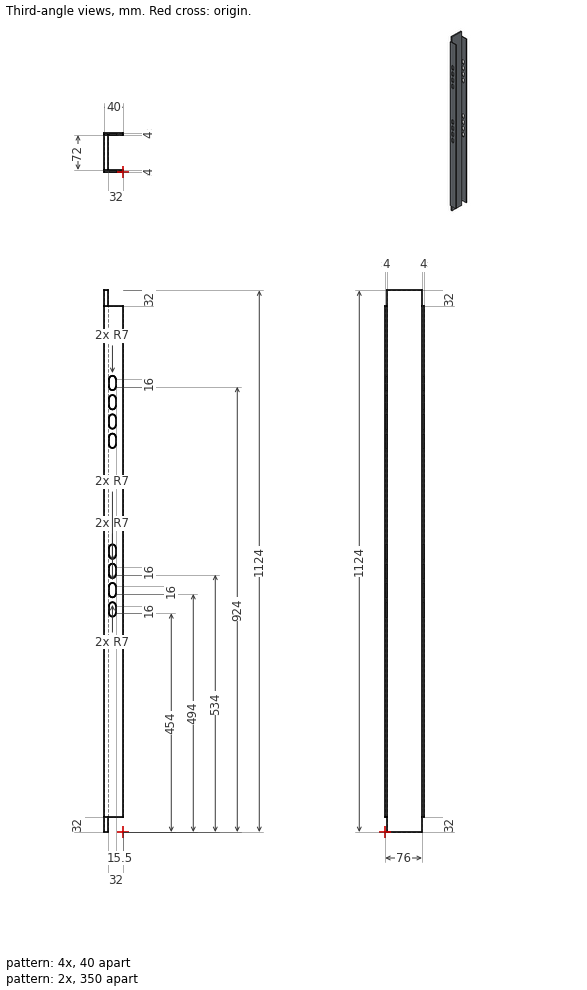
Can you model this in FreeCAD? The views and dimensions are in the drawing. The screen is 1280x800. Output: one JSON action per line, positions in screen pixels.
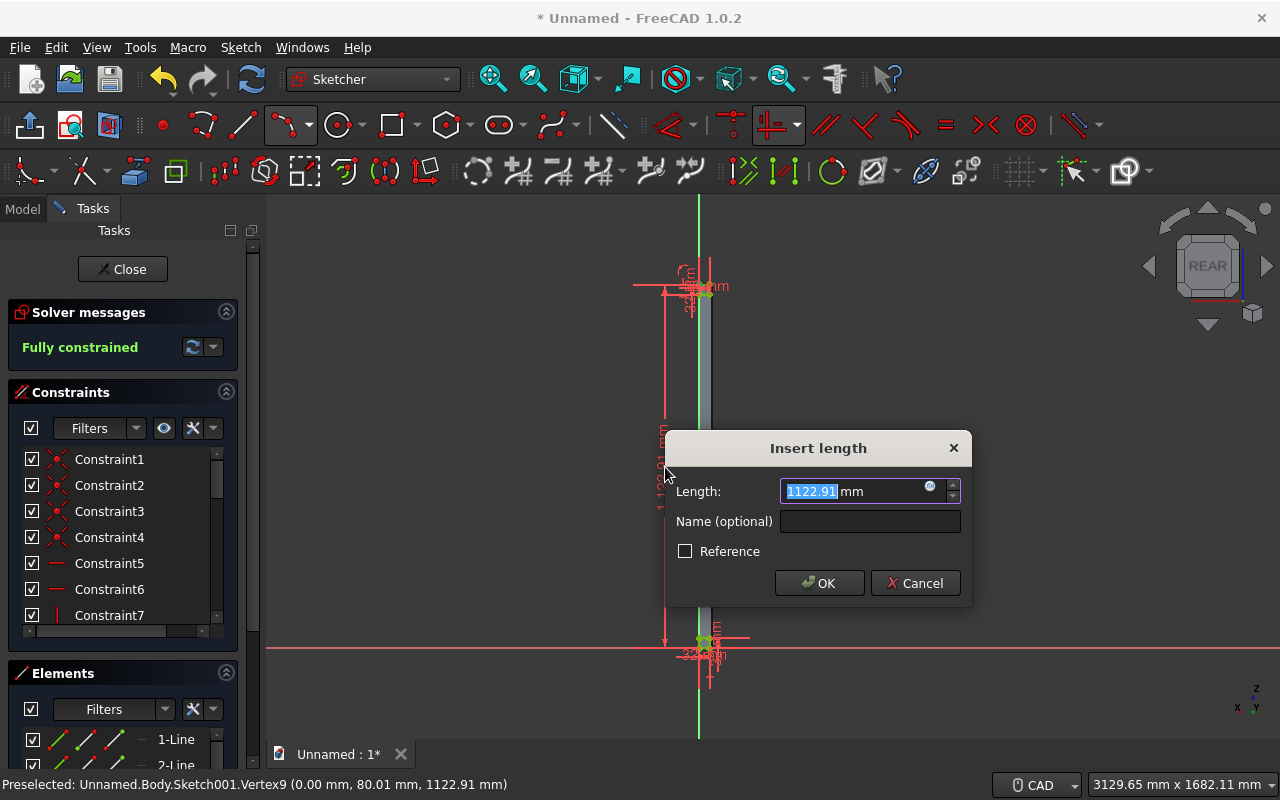
{"action": "type", "text": "1124"}
{"action": "key", "text": "Return"}
{"action": "key", "text": "Escape"}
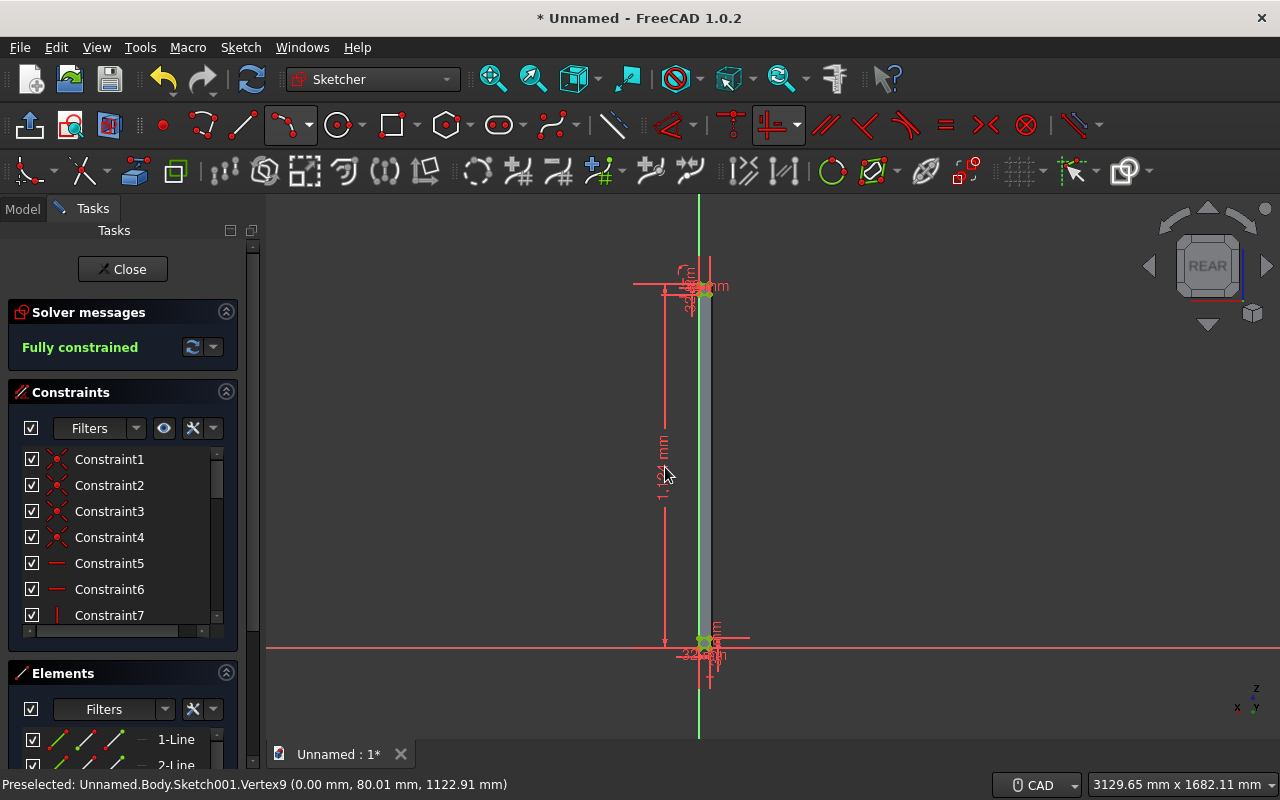
{"action": "left_click", "coordinate": [123, 269]}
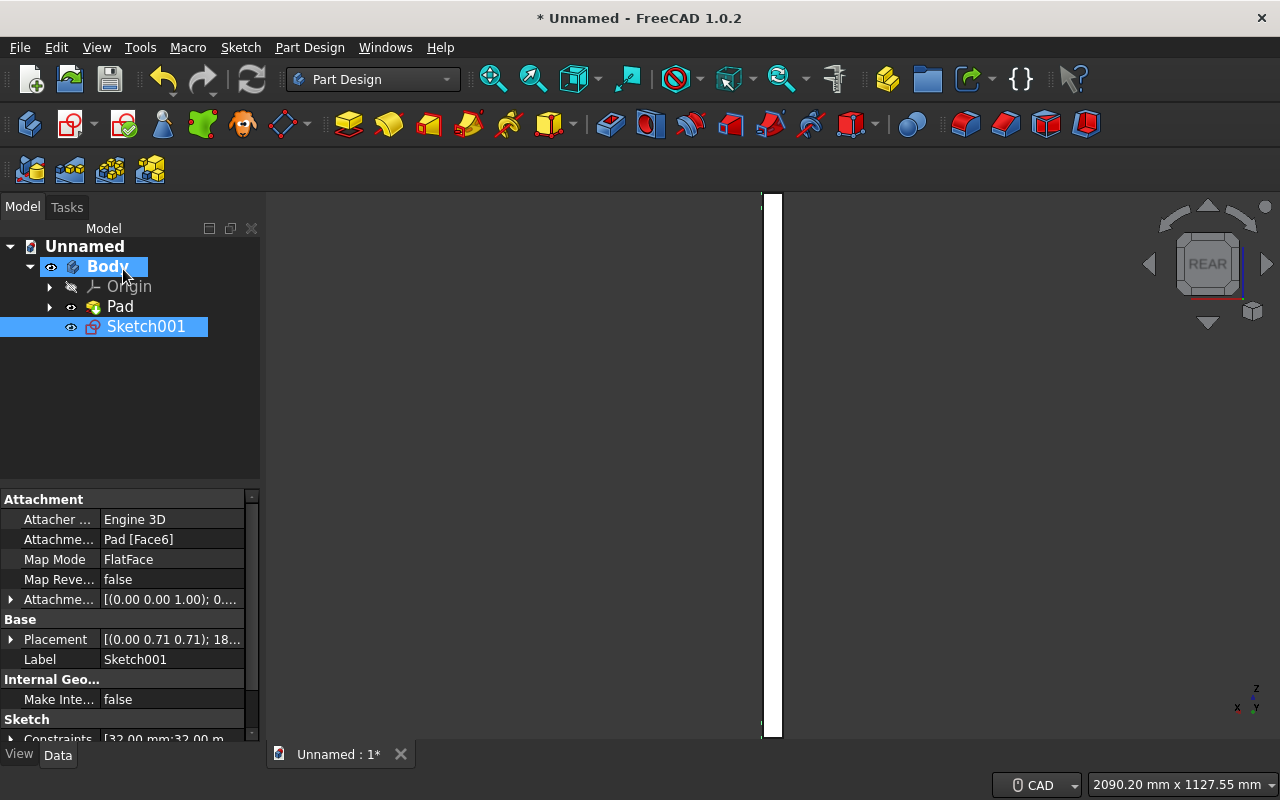
{"action": "left_click", "coordinate": [612, 124]}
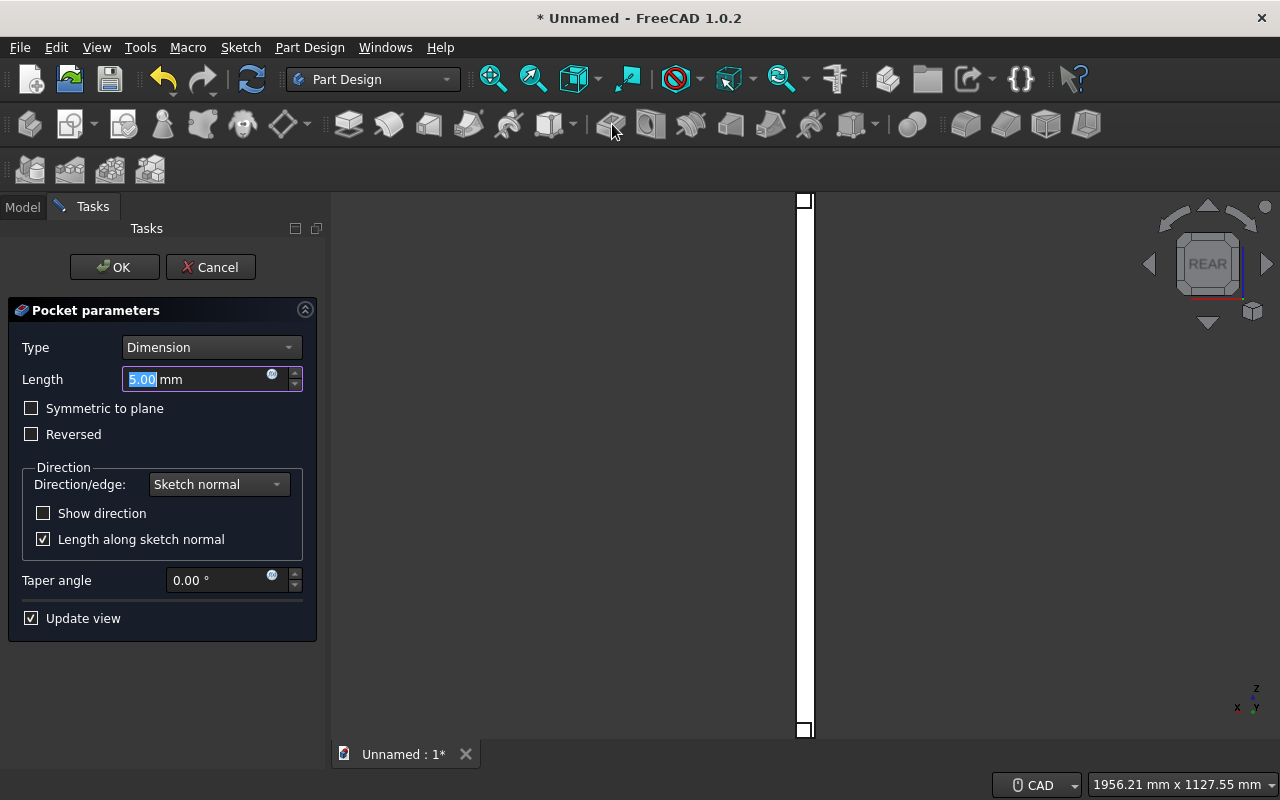
{"action": "left_click", "coordinate": [212, 348]}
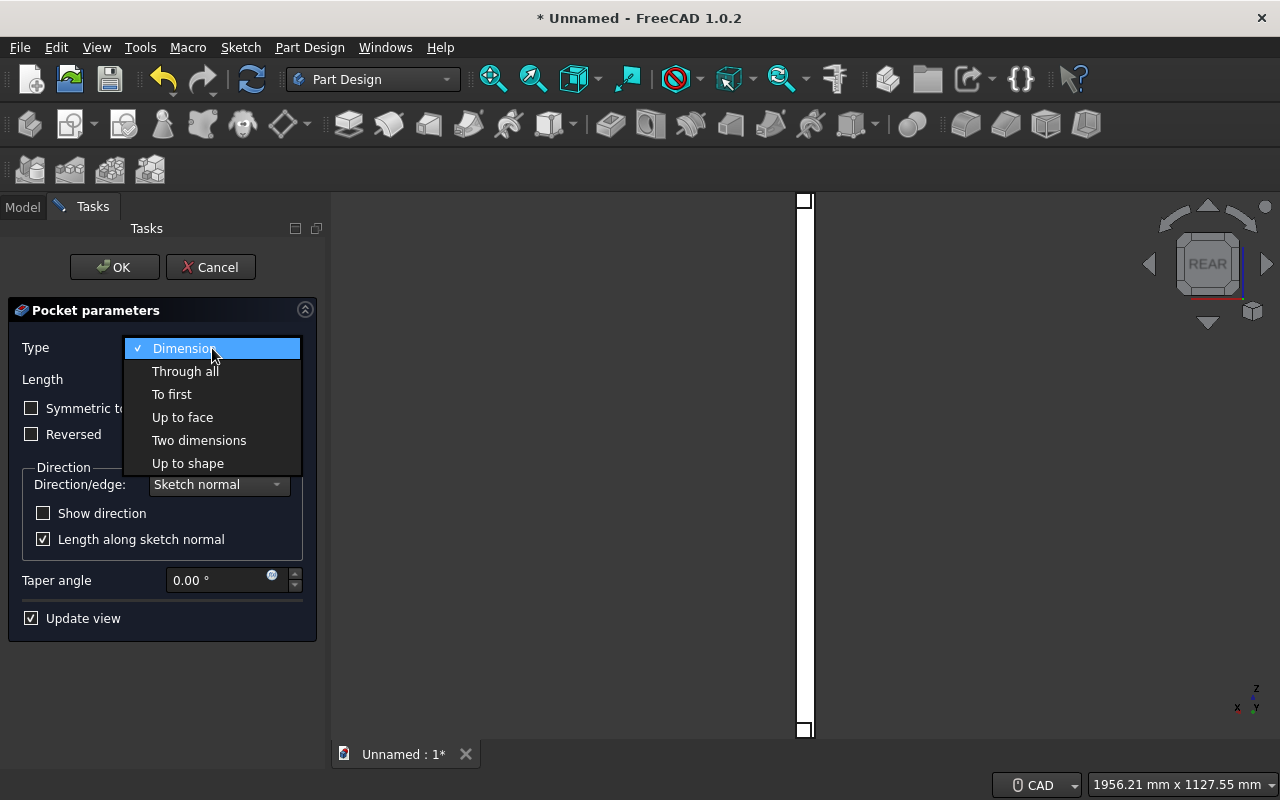
{"action": "left_click", "coordinate": [212, 372]}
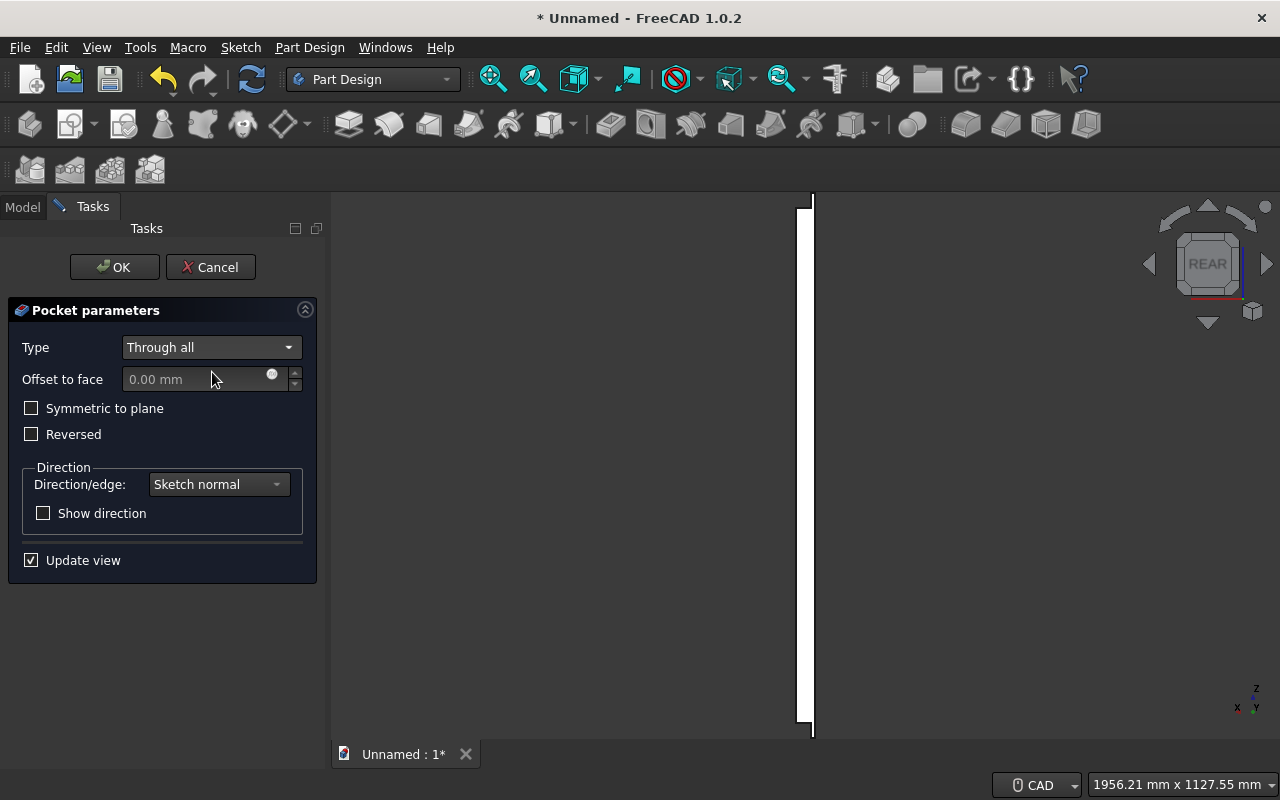
{"action": "left_click", "coordinate": [115, 267]}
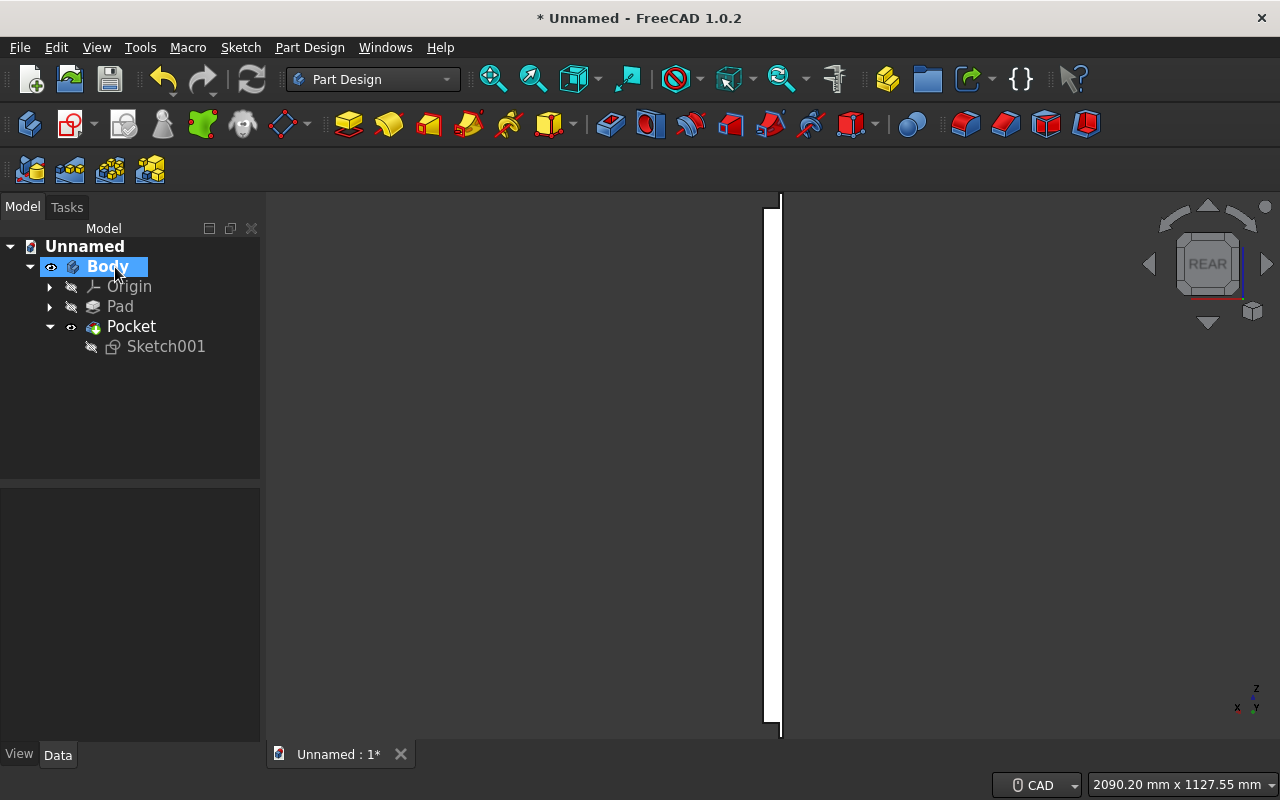
{"action": "key", "text": "0"}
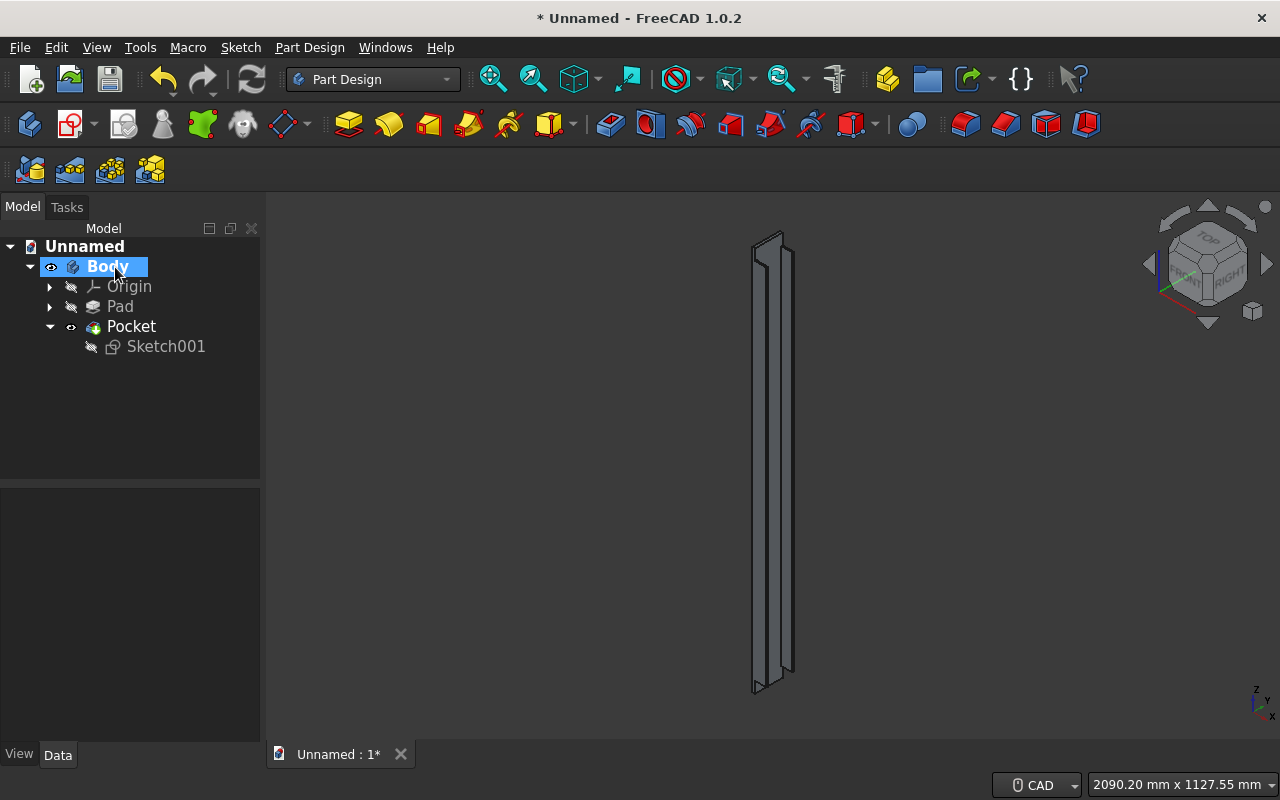
{"action": "key", "text": "3"}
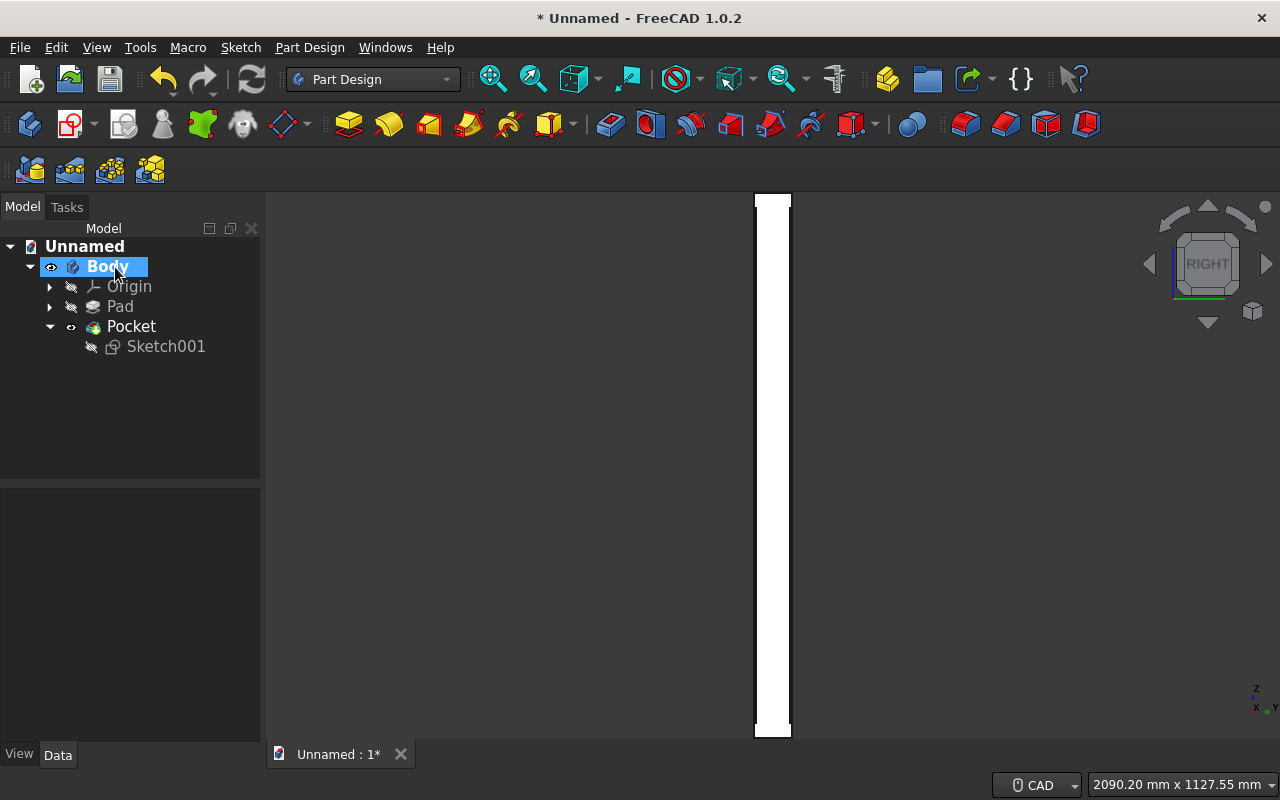
{"action": "left_click", "coordinate": [773, 231]}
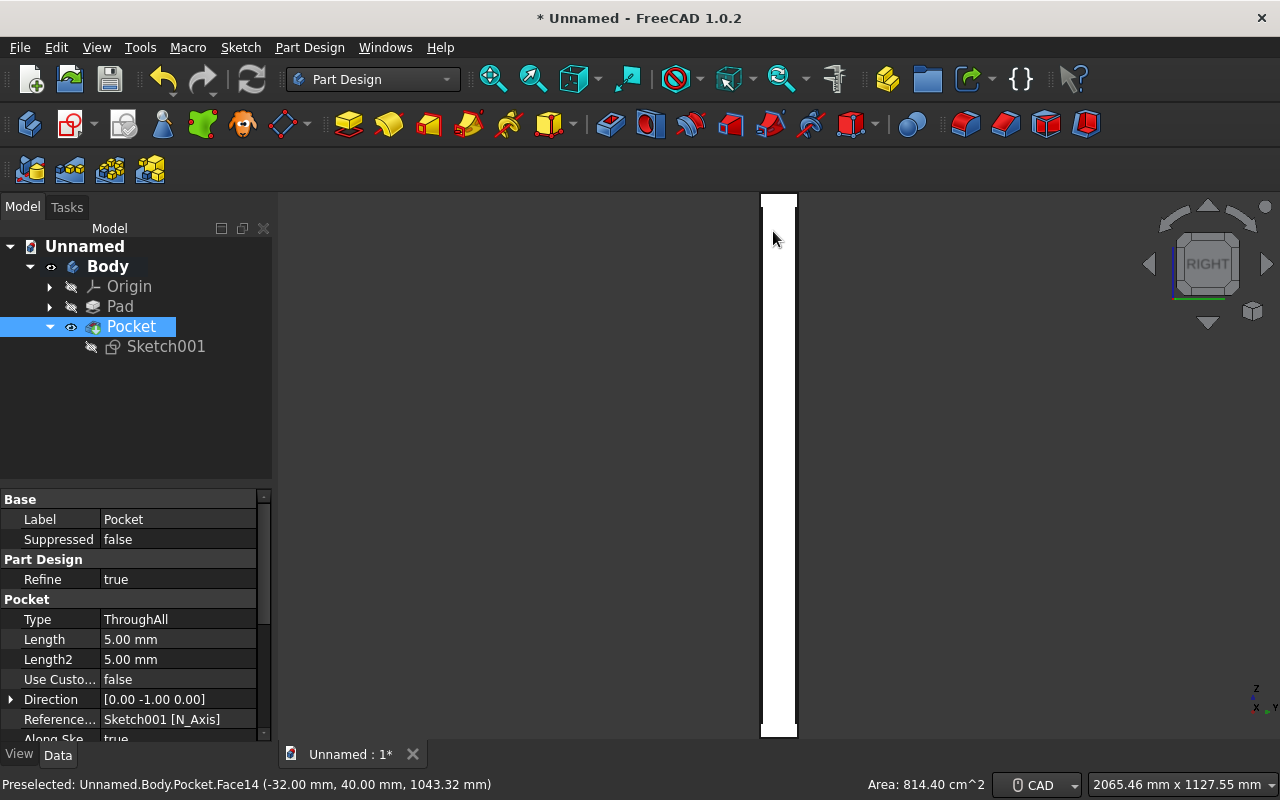
{"action": "left_click", "coordinate": [70, 124]}